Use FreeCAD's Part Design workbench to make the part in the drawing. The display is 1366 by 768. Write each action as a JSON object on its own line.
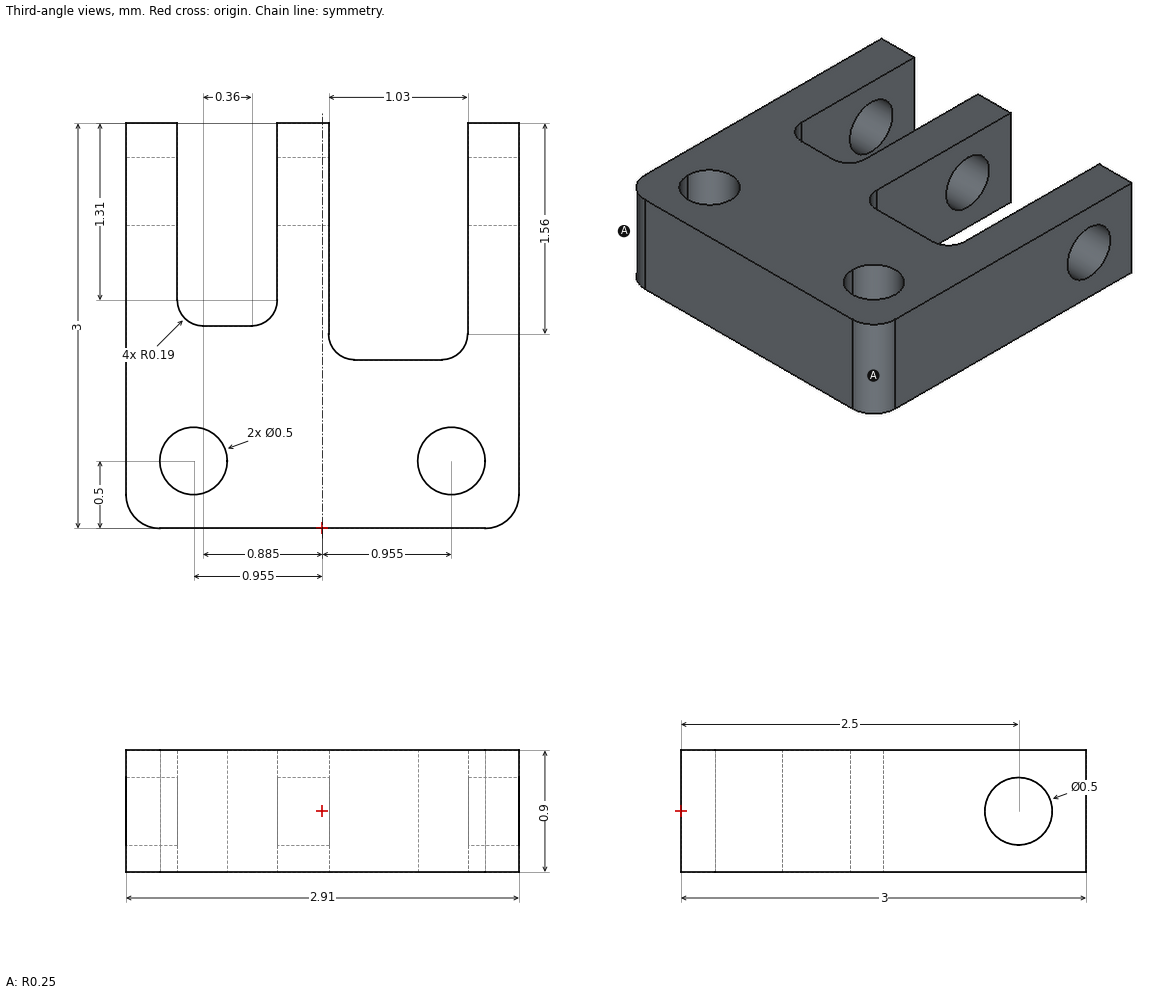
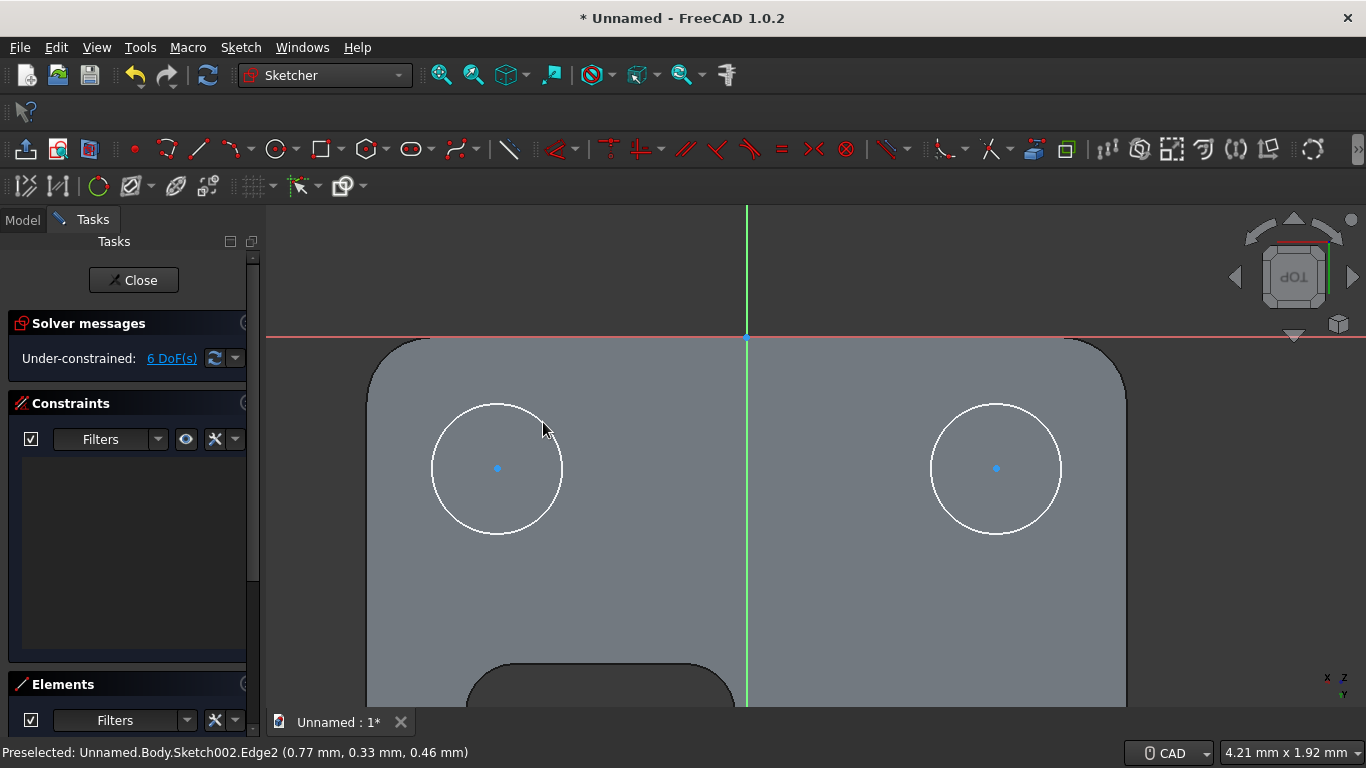
{"action": "left_click", "coordinate": [1042, 423]}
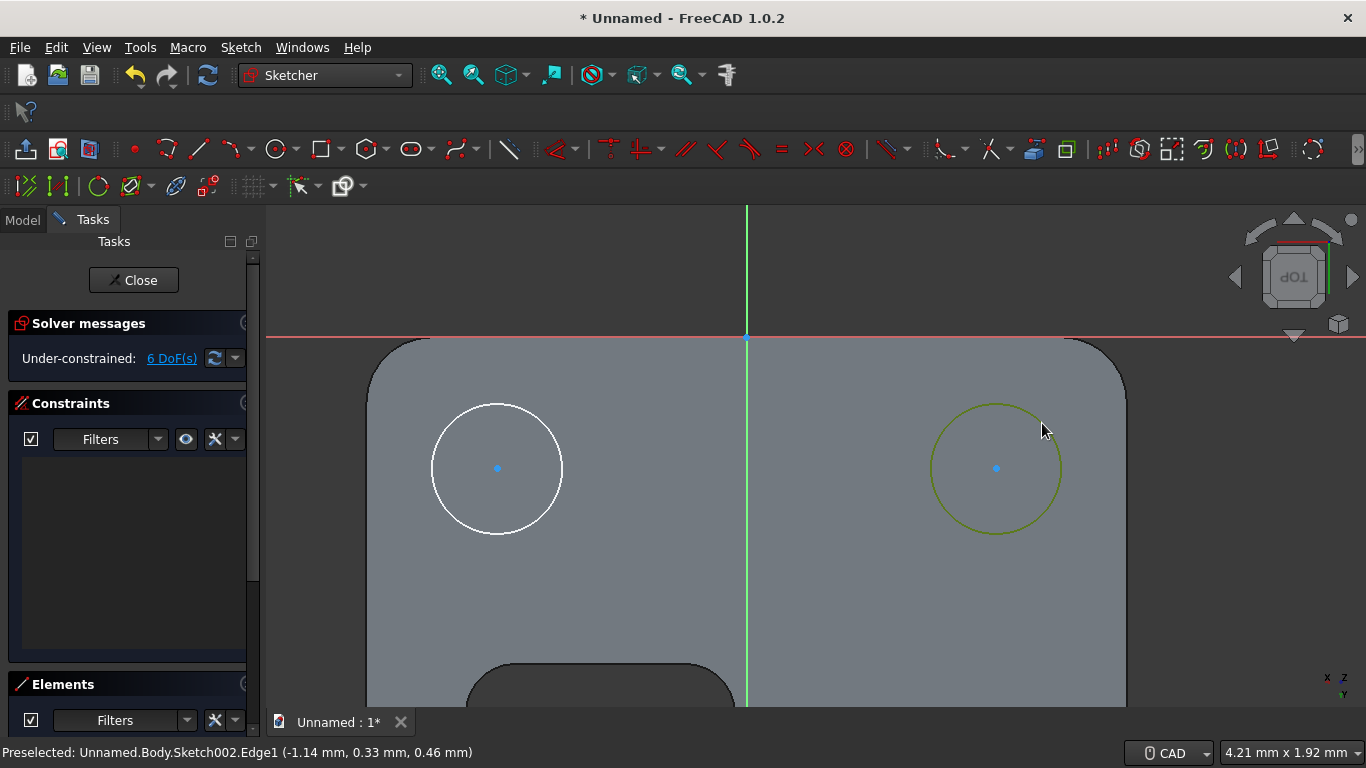
{"action": "left_click", "coordinate": [543, 423]}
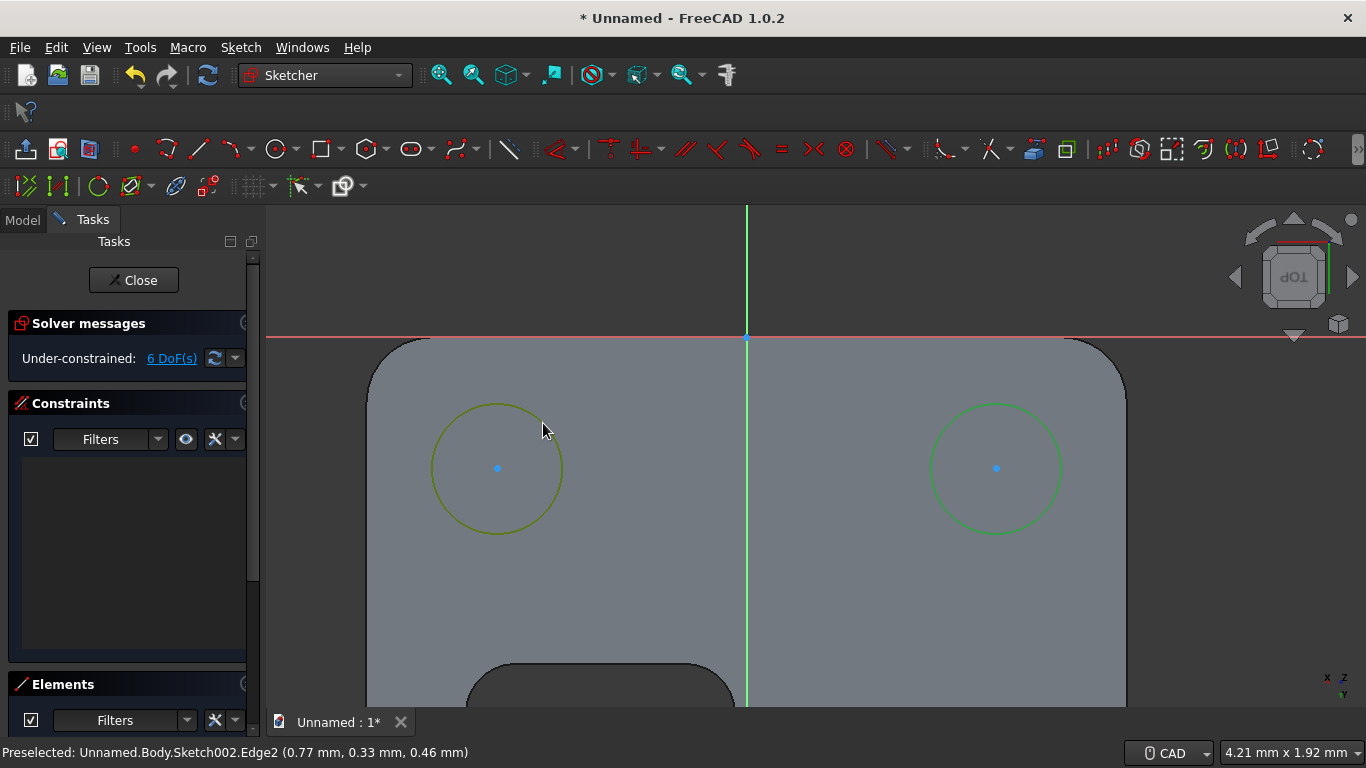
{"action": "key", "text": "e"}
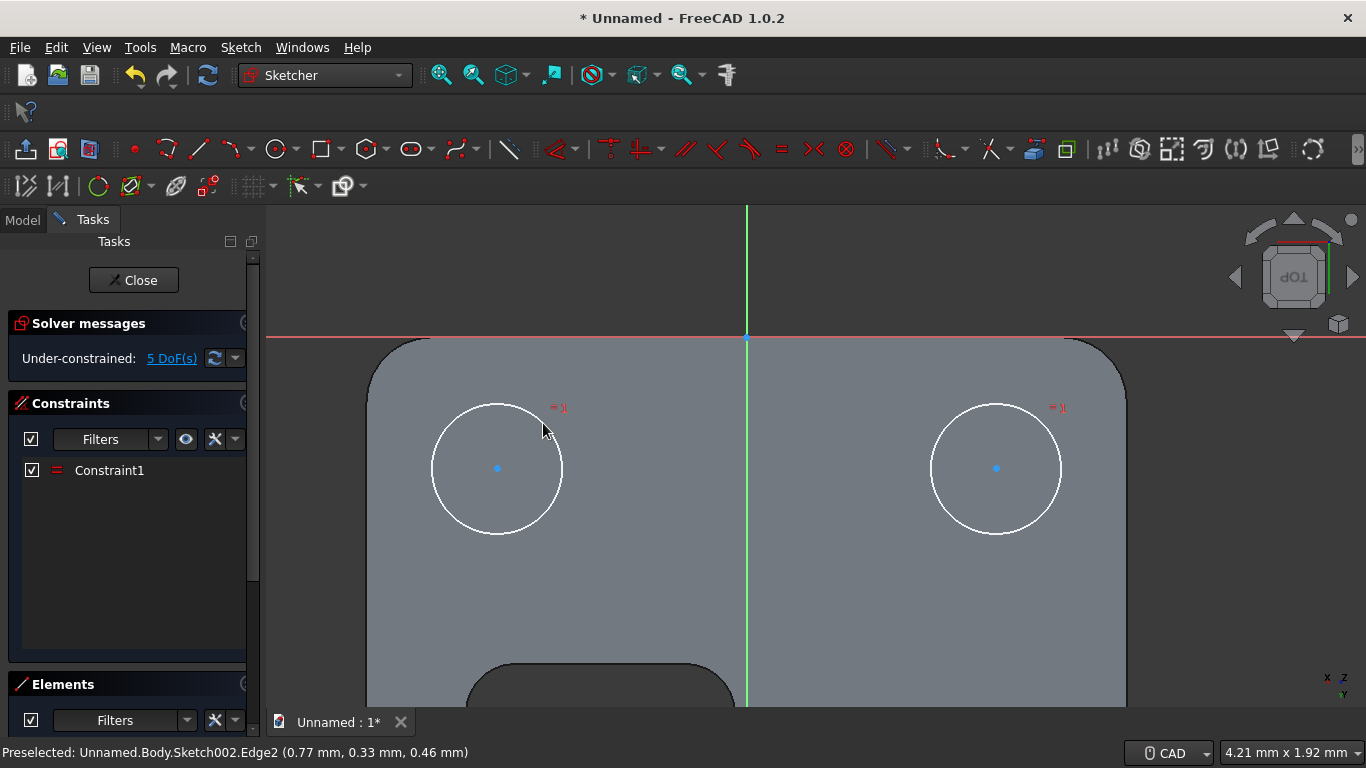
{"action": "left_click", "coordinate": [996, 469]}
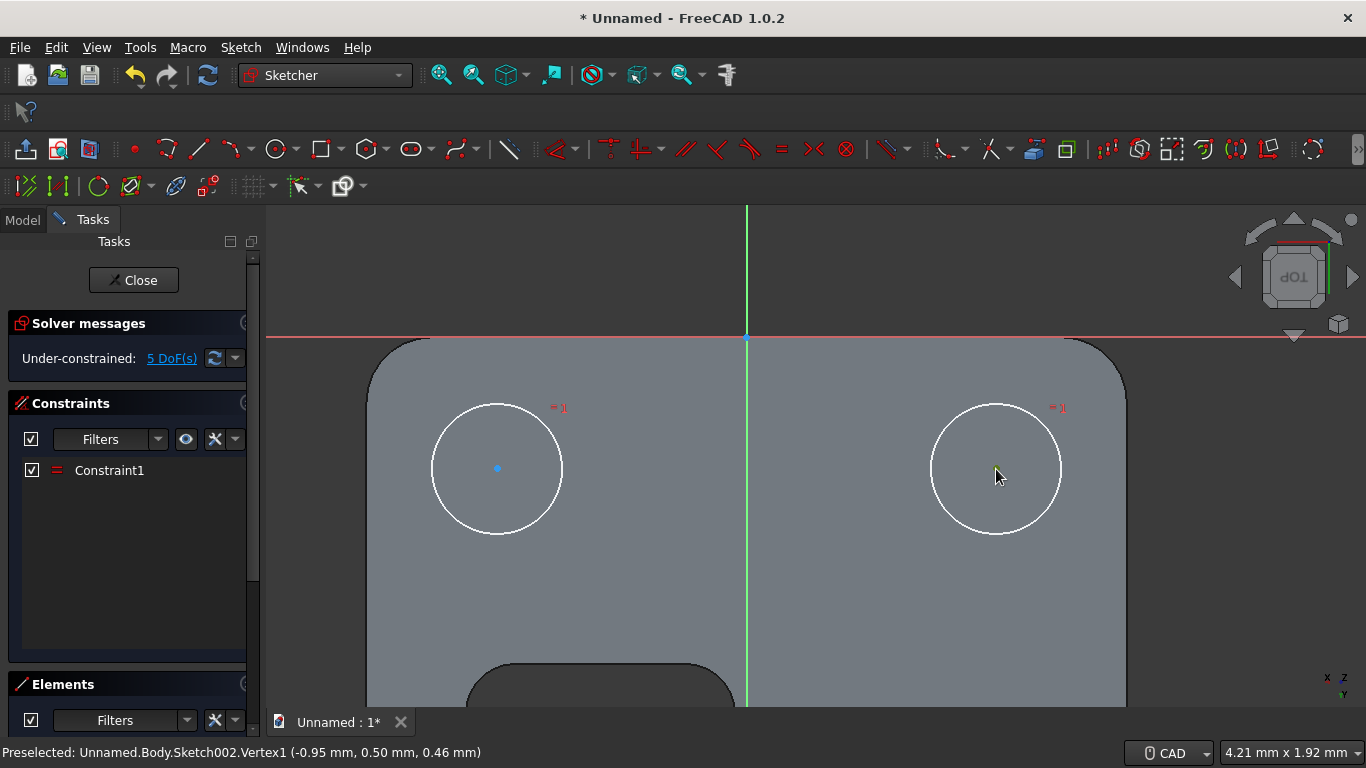
{"action": "left_click", "coordinate": [497, 469]}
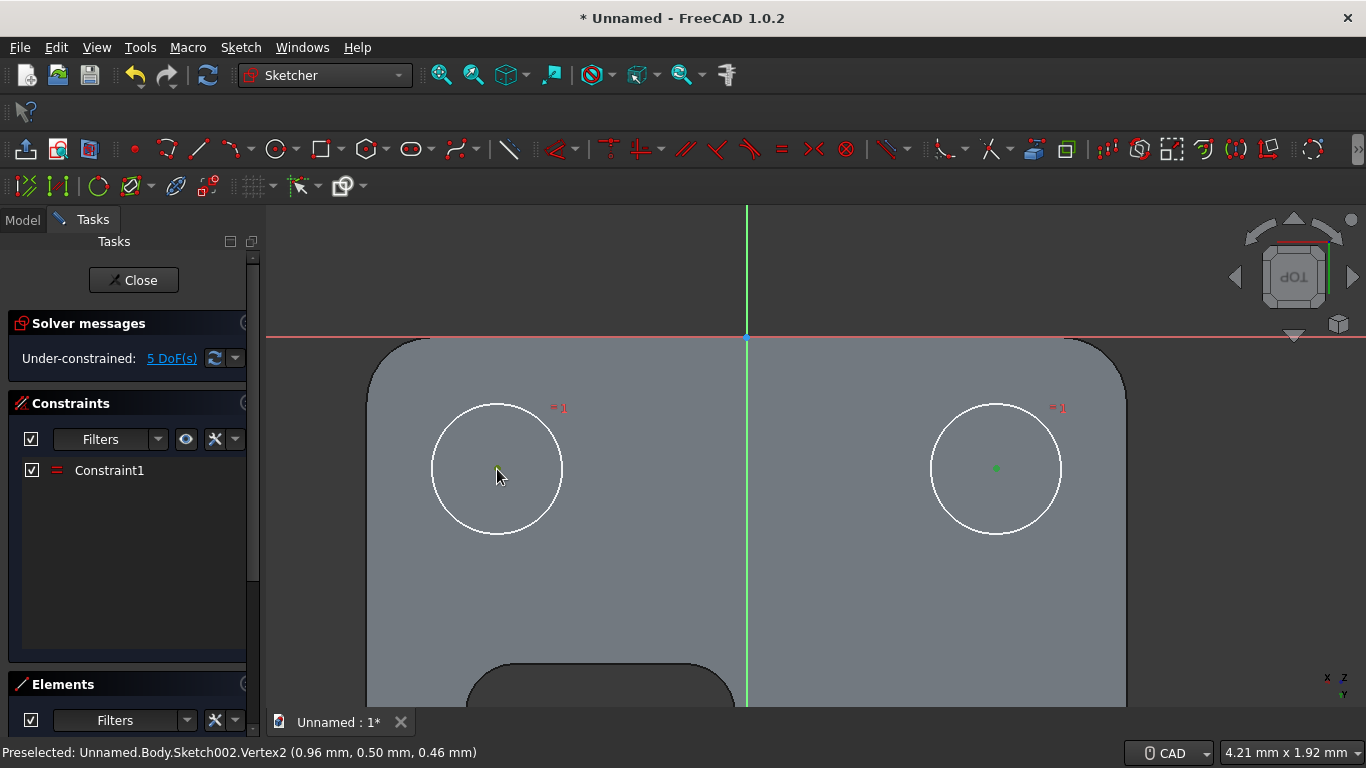
{"action": "key", "text": "h"}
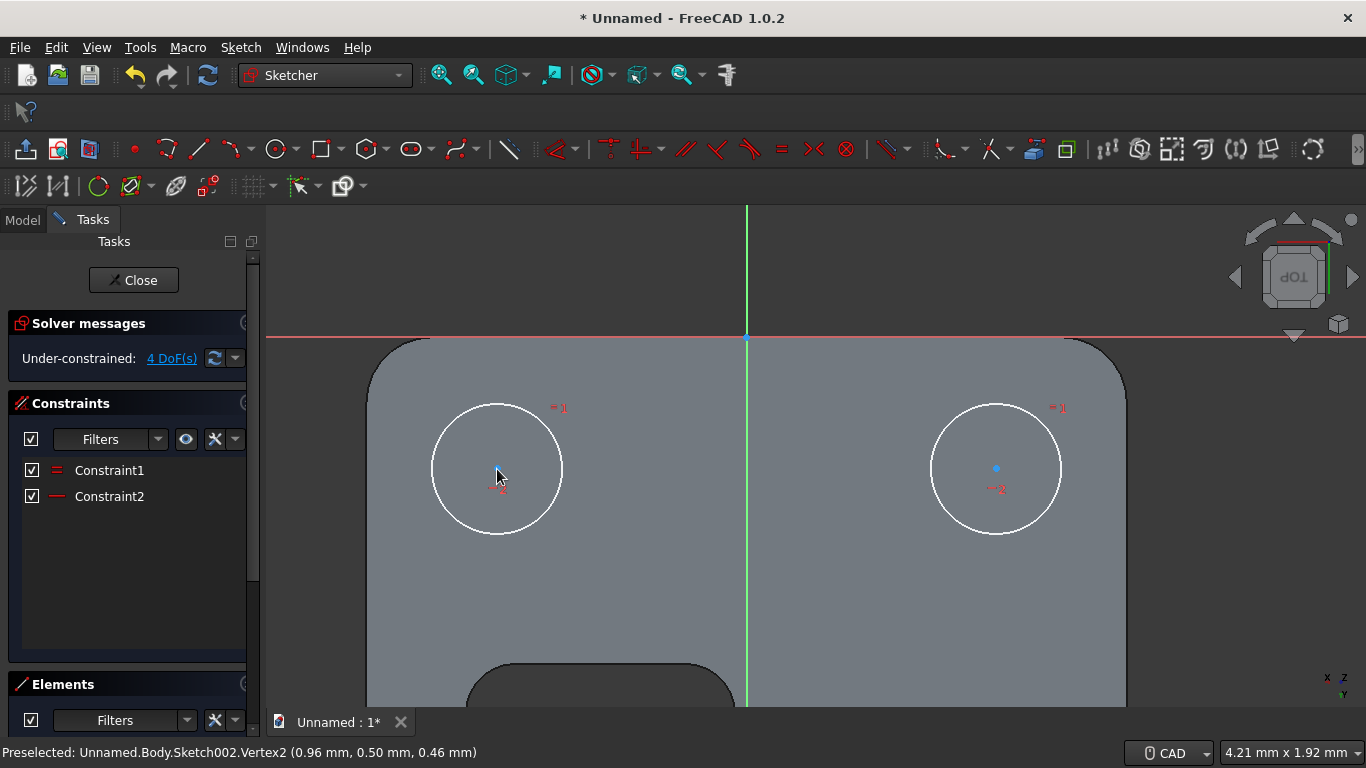
{"action": "key", "text": "d"}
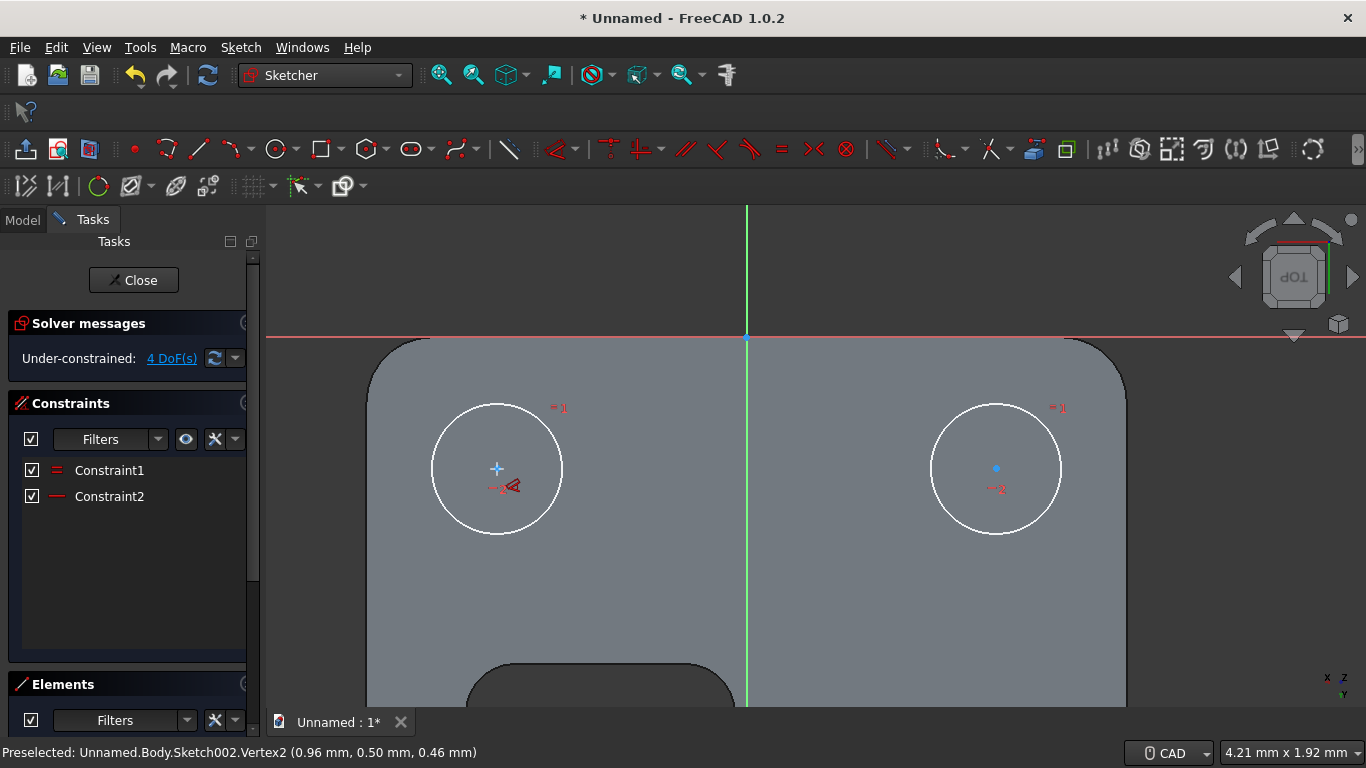
{"action": "left_click", "coordinate": [1042, 423]}
{"action": "left_click", "coordinate": [1065, 400]}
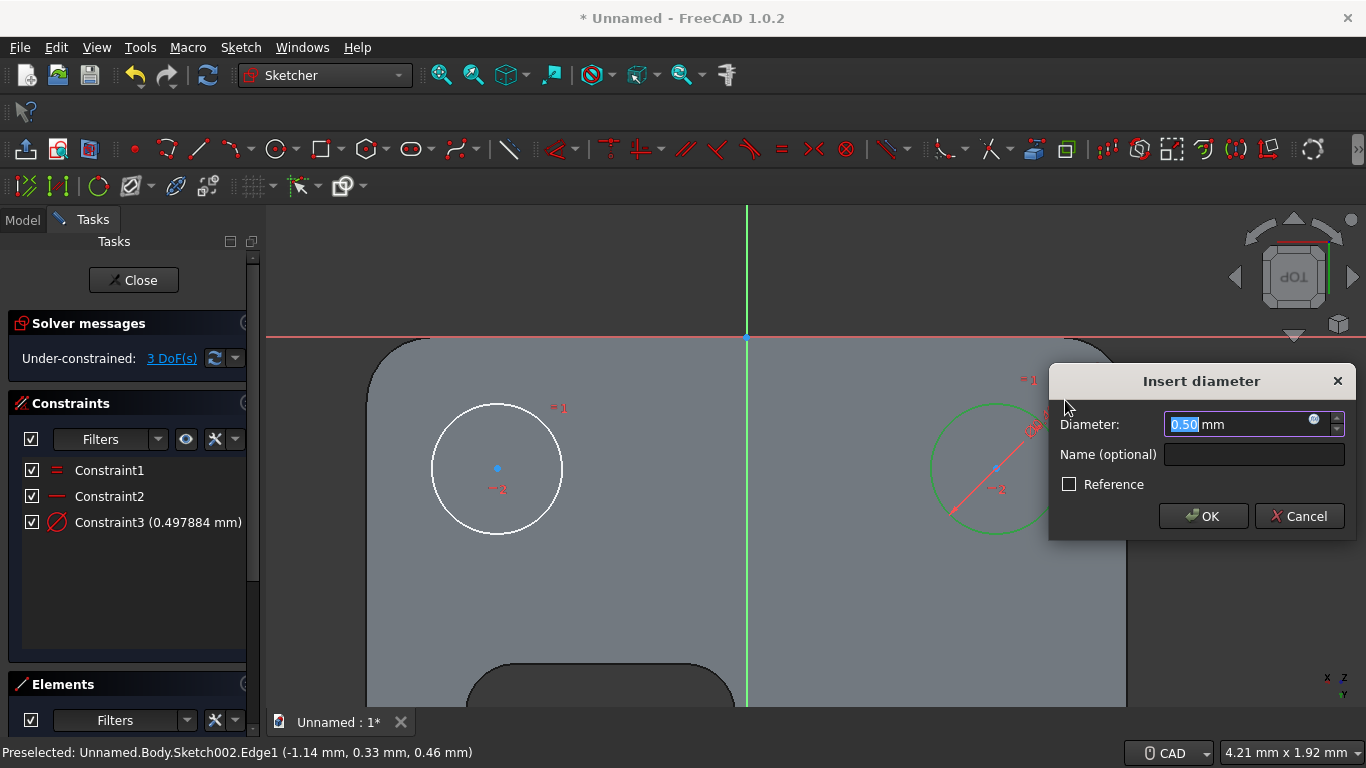
{"action": "type", "text": "0.5"}
{"action": "key", "text": "Return"}